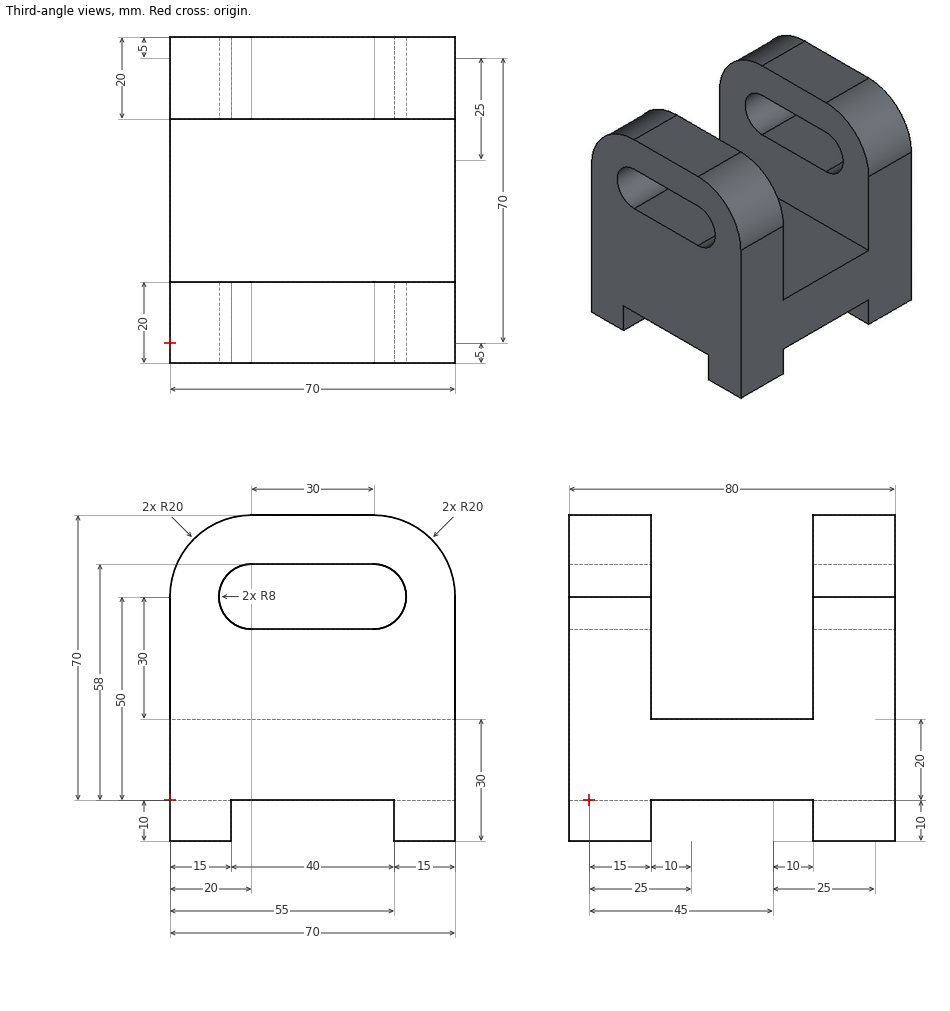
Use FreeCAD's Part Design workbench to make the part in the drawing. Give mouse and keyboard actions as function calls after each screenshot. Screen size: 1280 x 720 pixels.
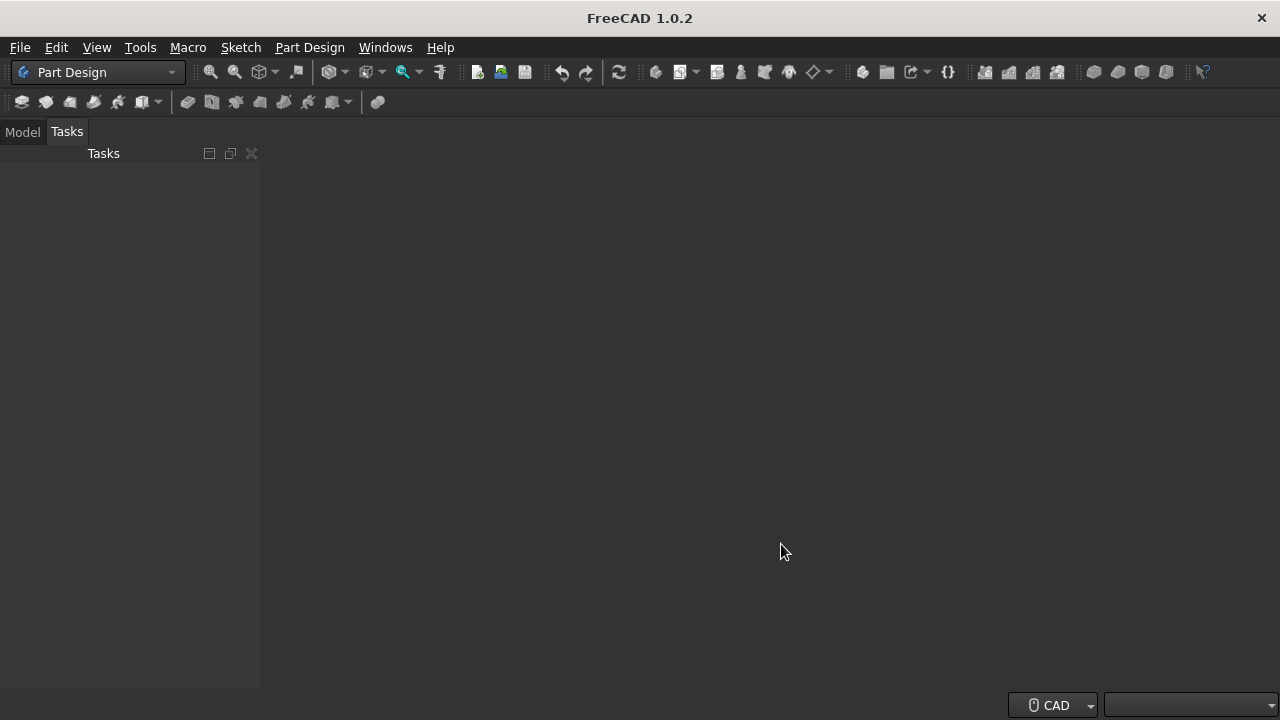
click(478, 72)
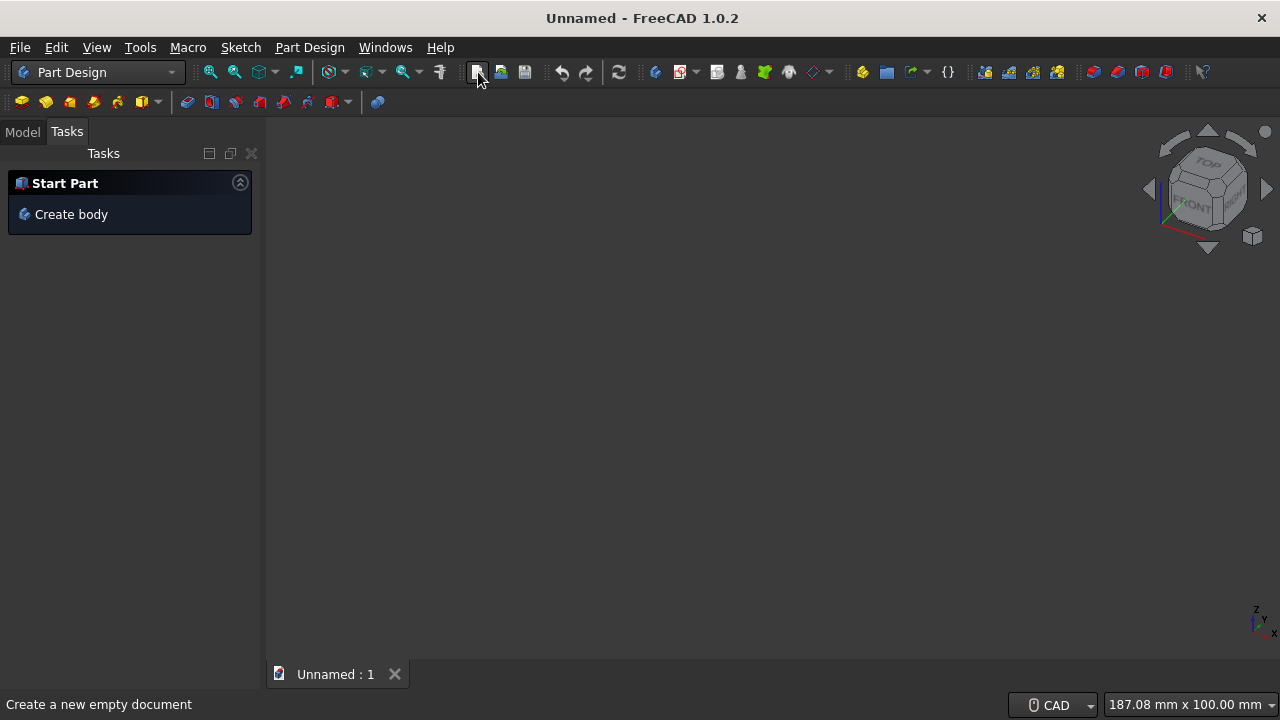
click(680, 72)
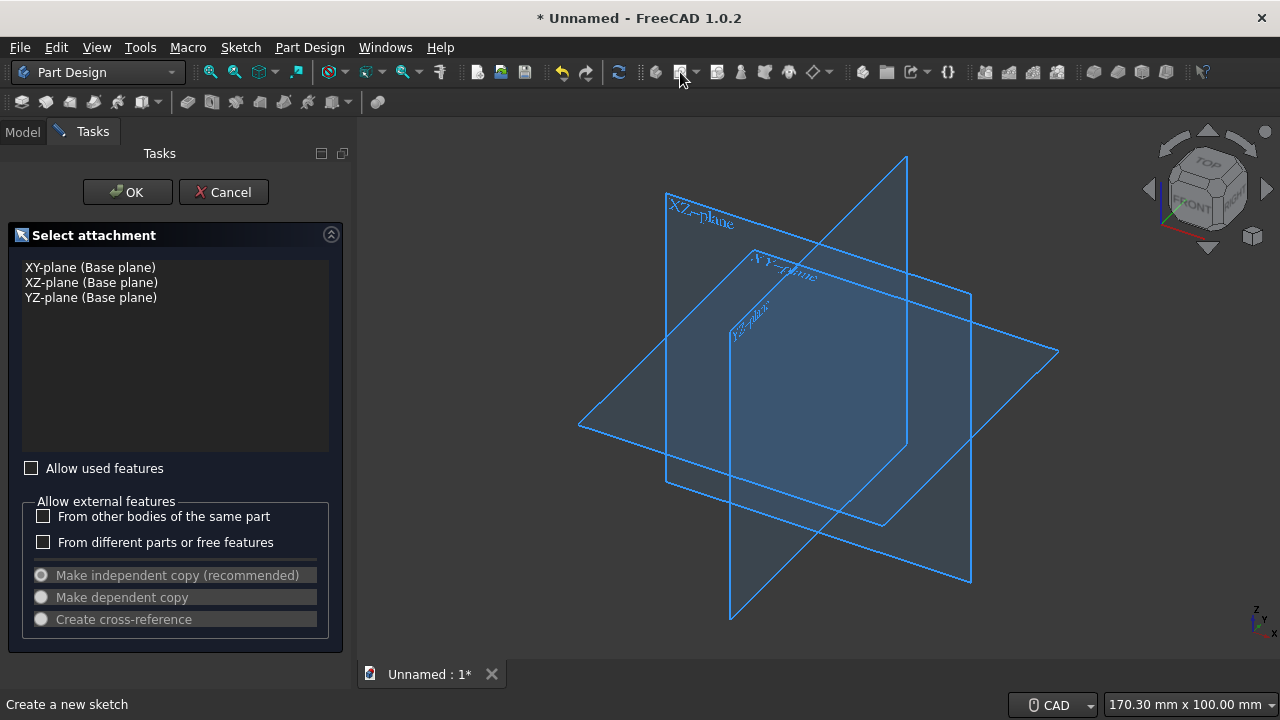
click(82, 268)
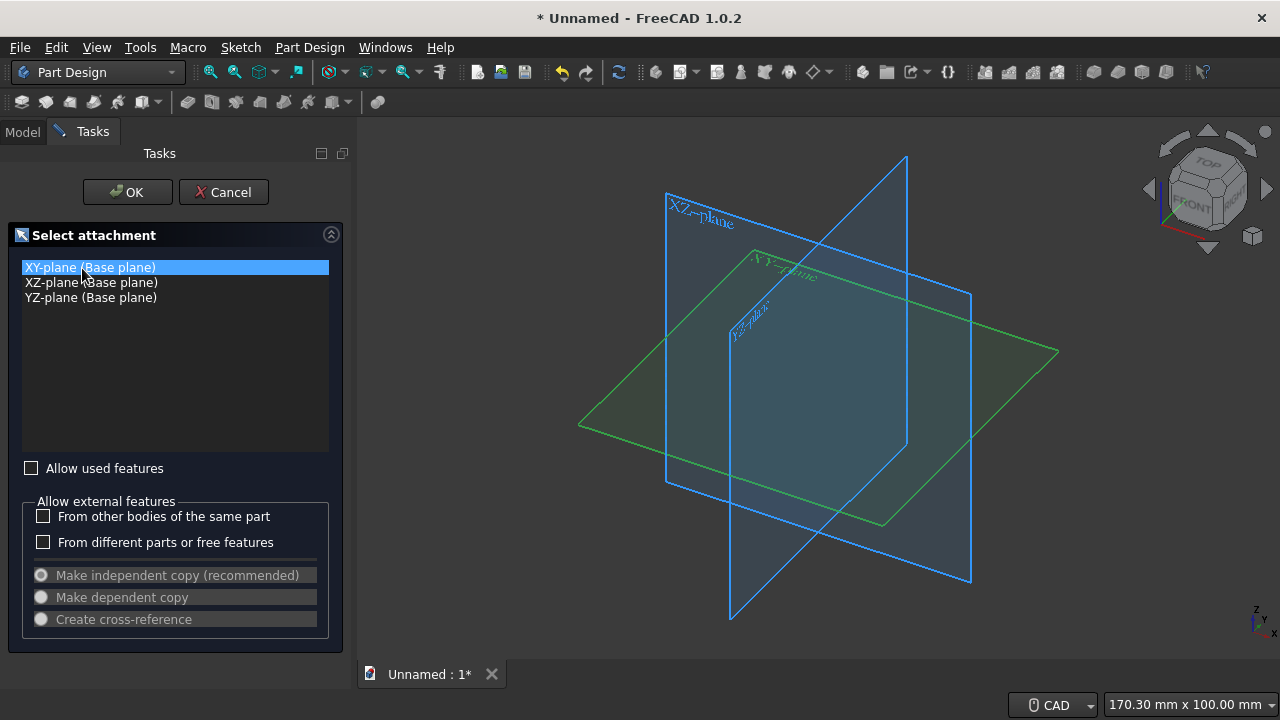
click(128, 192)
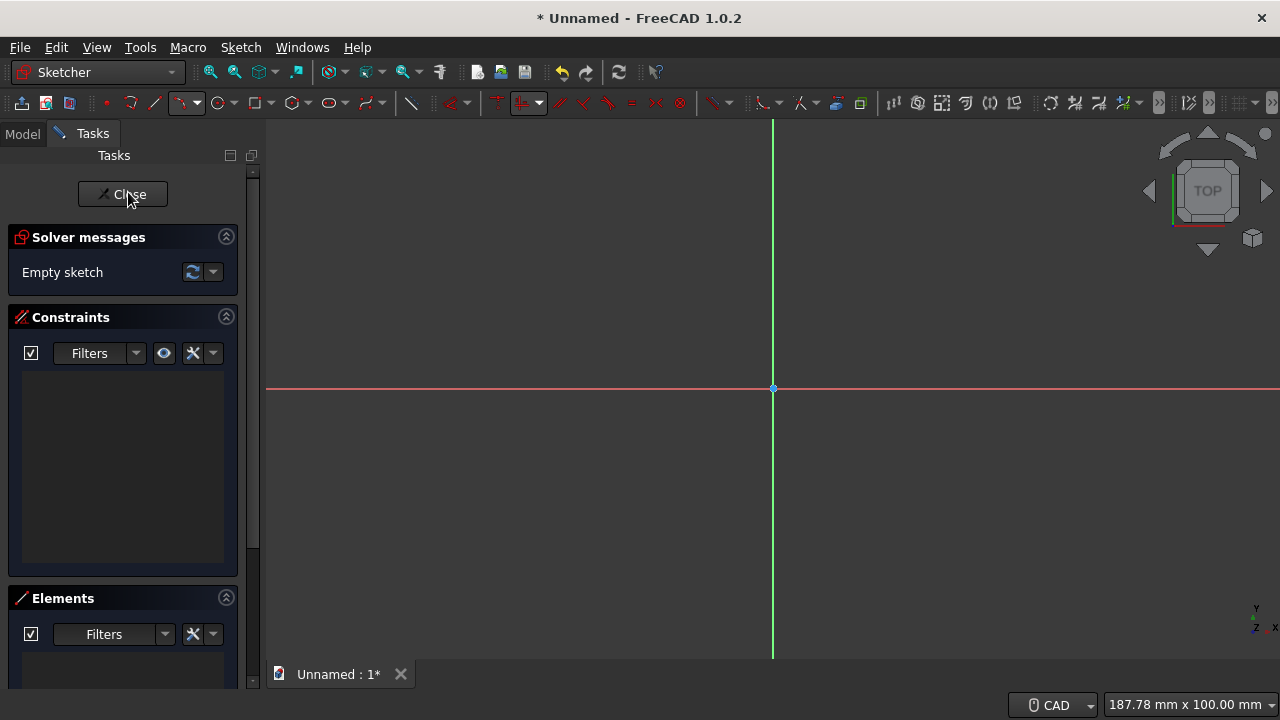
scroll(294, 631, down, 2)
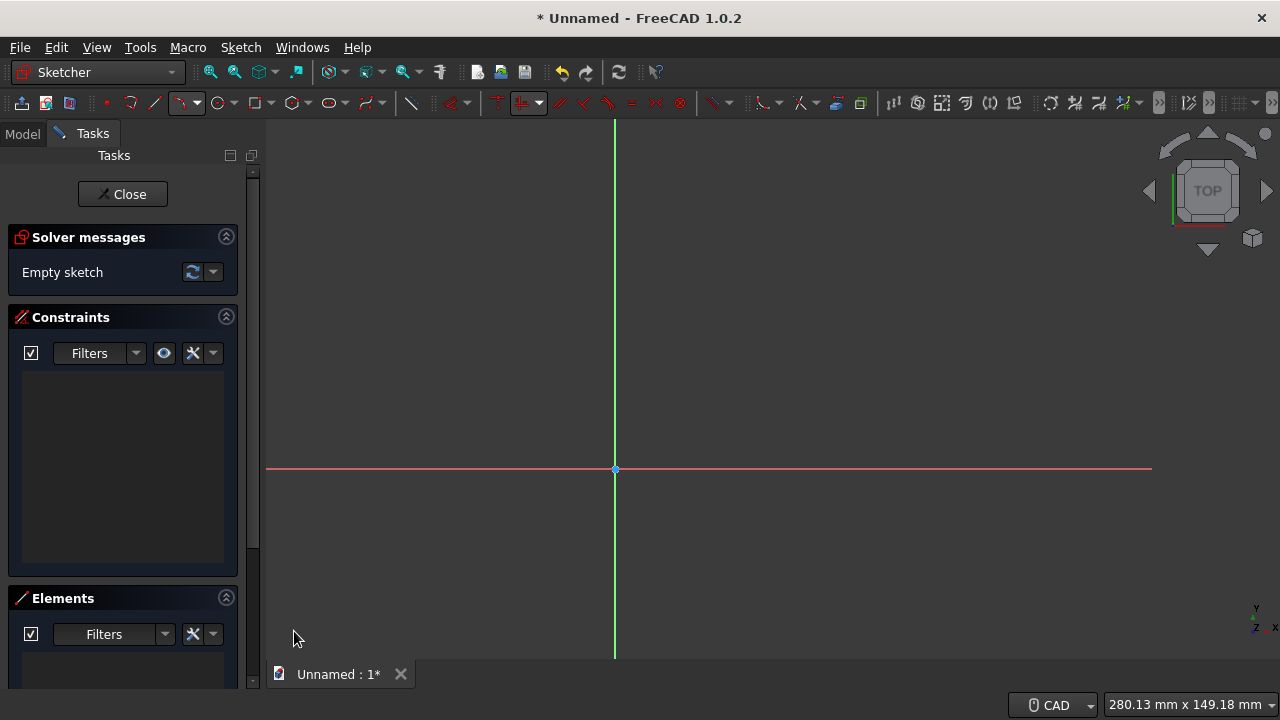
key(g)
key(r)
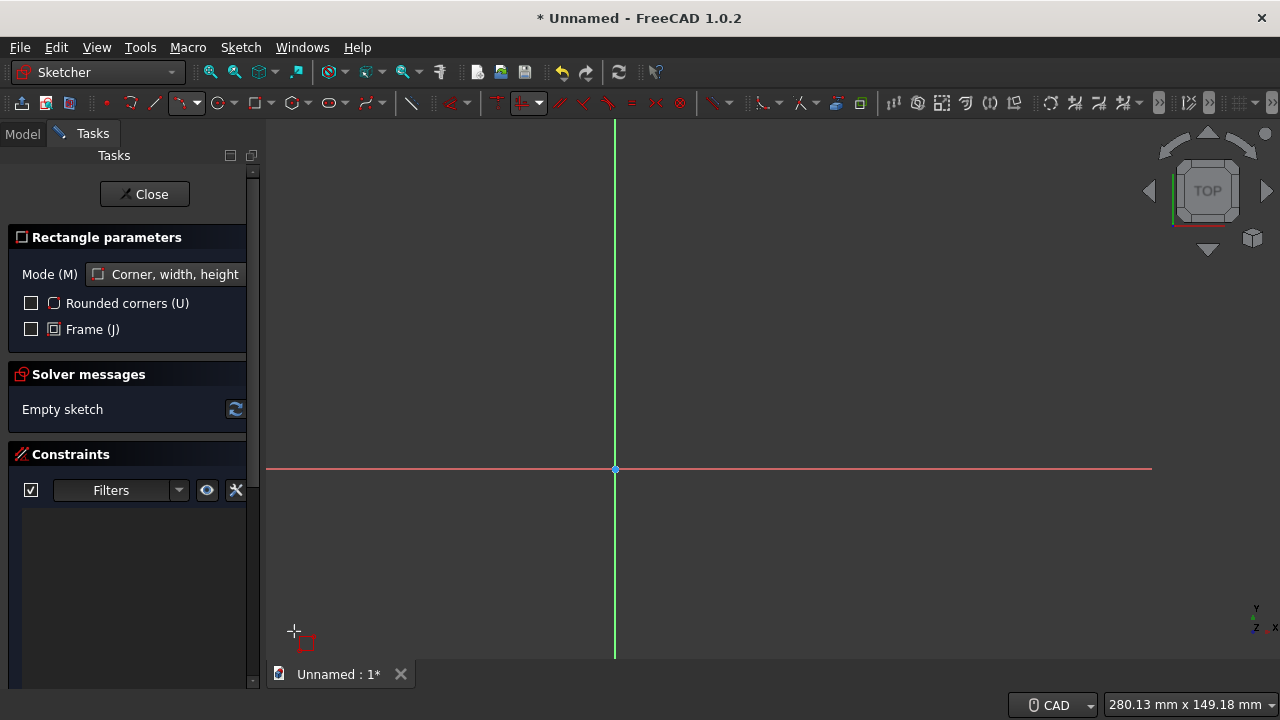
click(615, 469)
click(868, 216)
key(Escape)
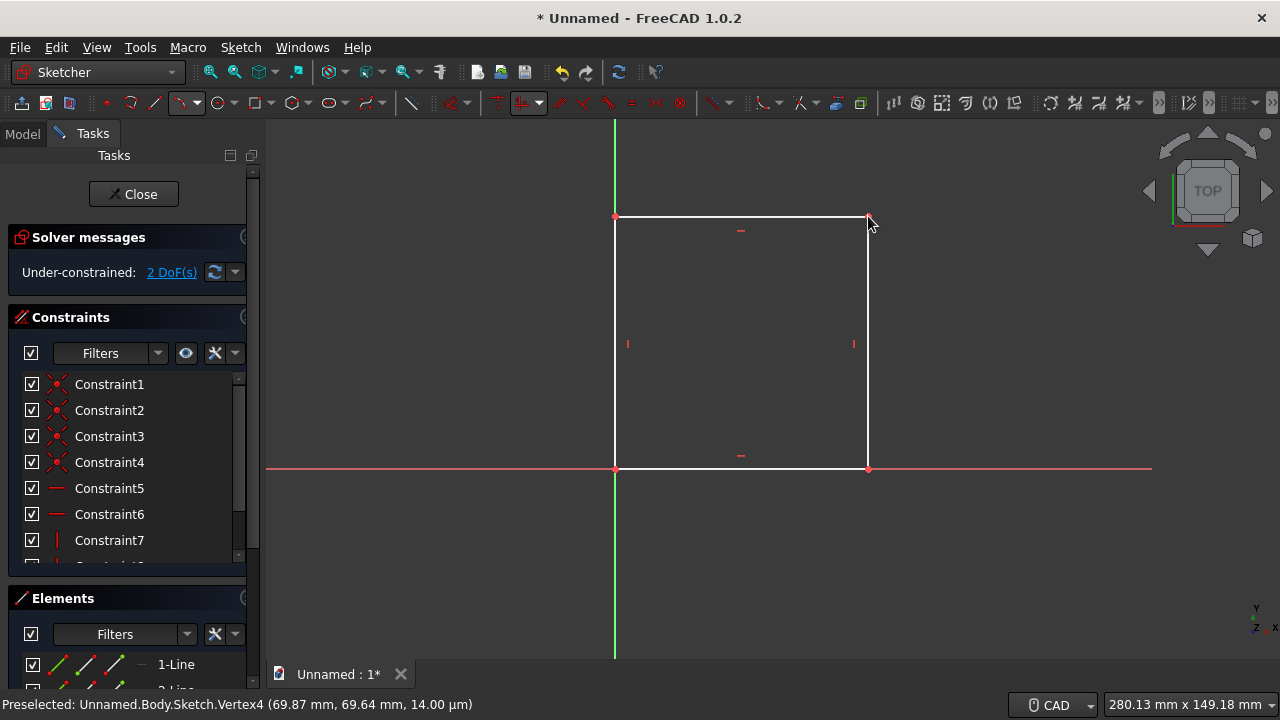
click(450, 104)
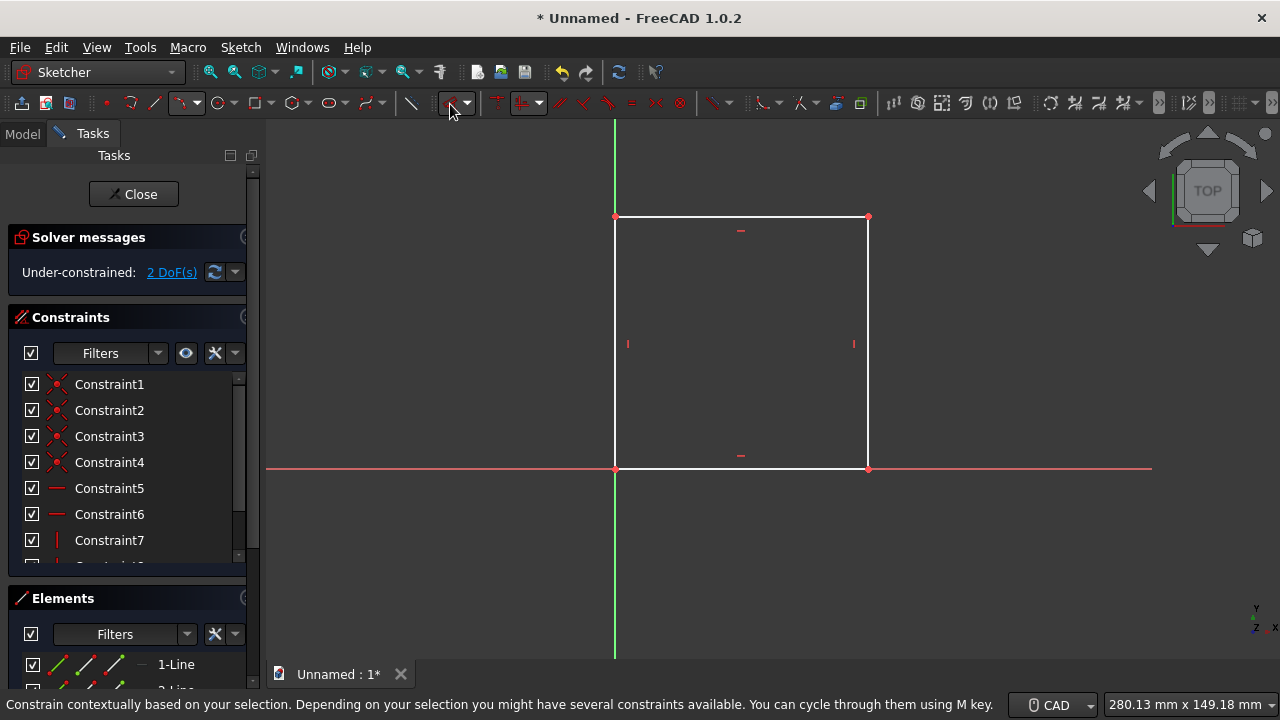
click(691, 469)
click(742, 503)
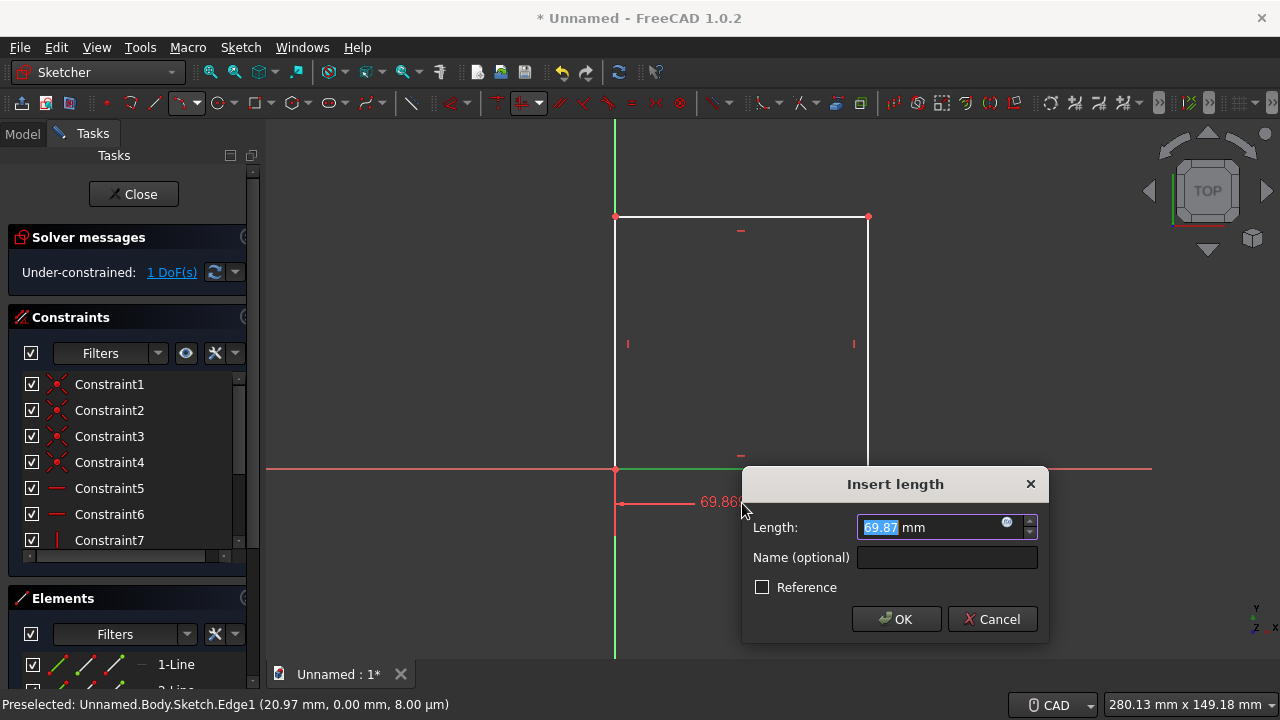
text(70)
key(Return)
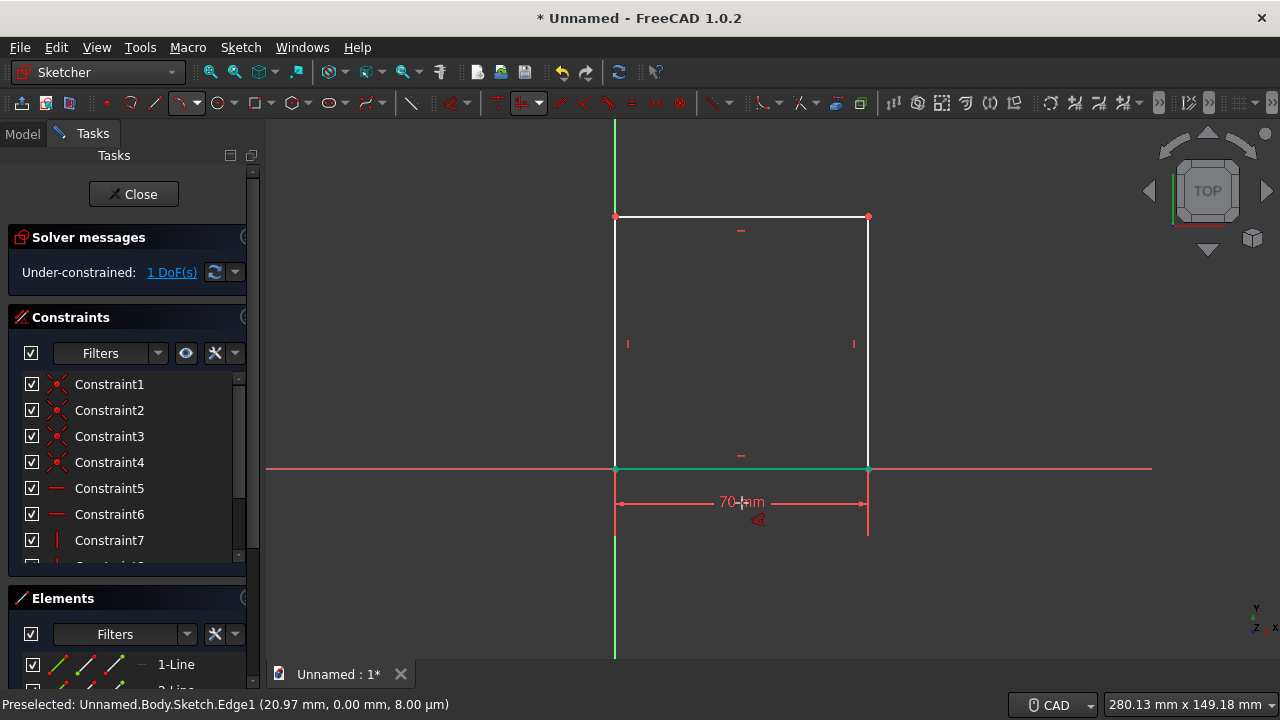
click(868, 393)
click(902, 343)